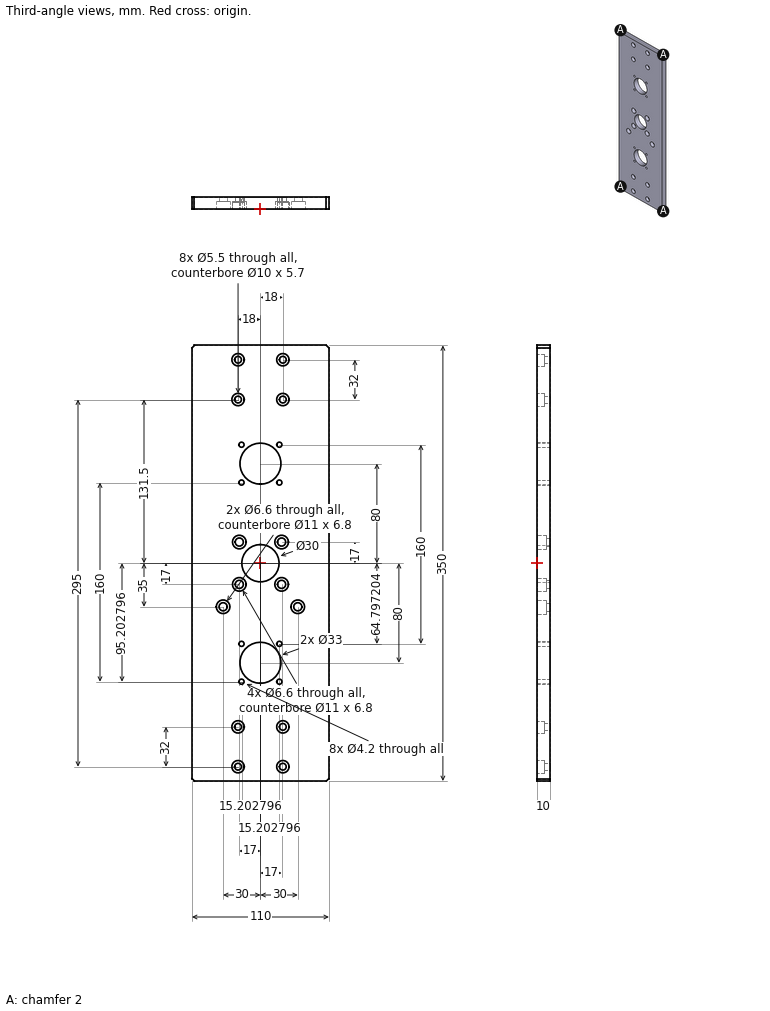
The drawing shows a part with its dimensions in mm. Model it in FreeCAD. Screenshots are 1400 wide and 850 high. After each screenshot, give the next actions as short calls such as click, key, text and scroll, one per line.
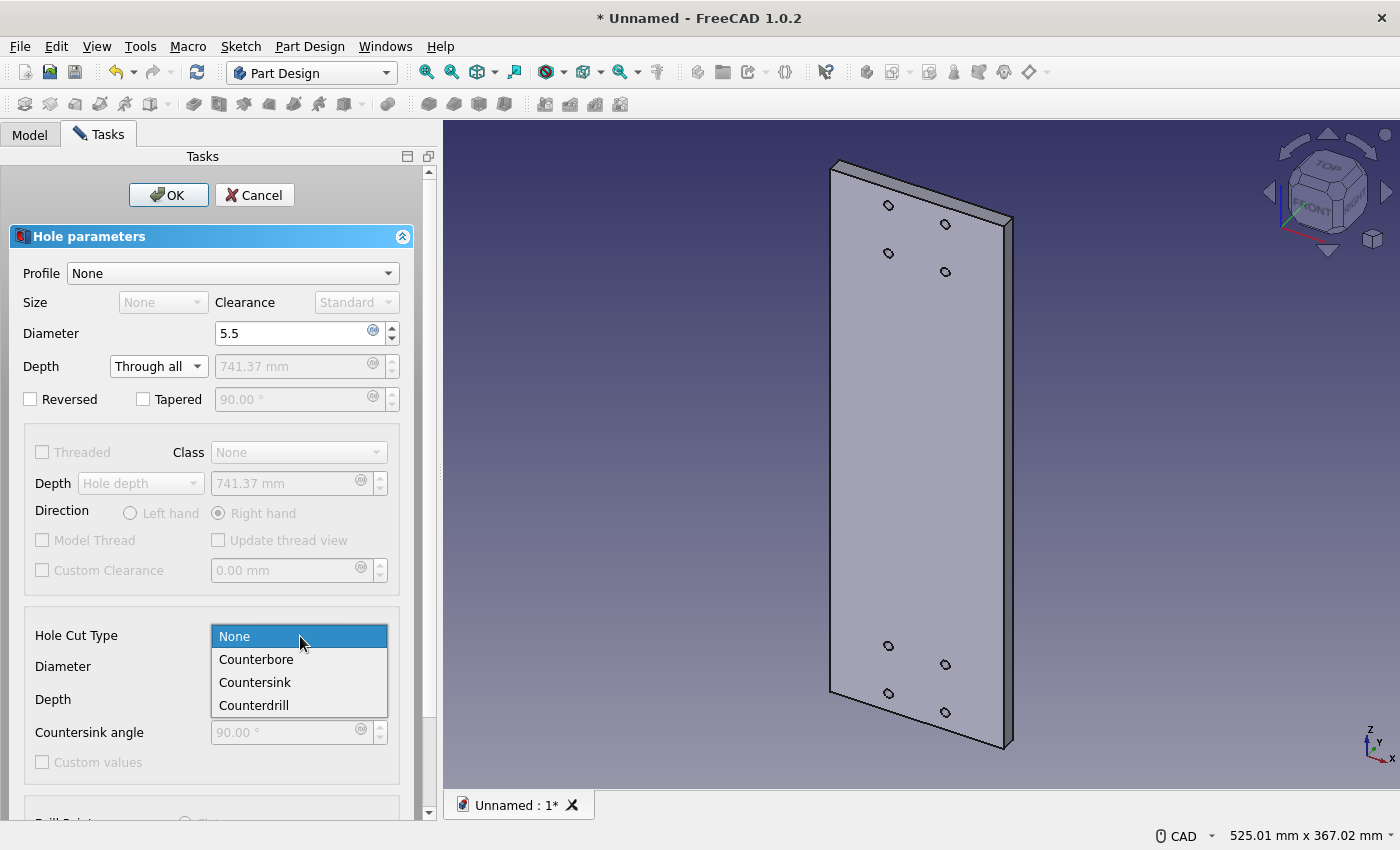
click(298, 660)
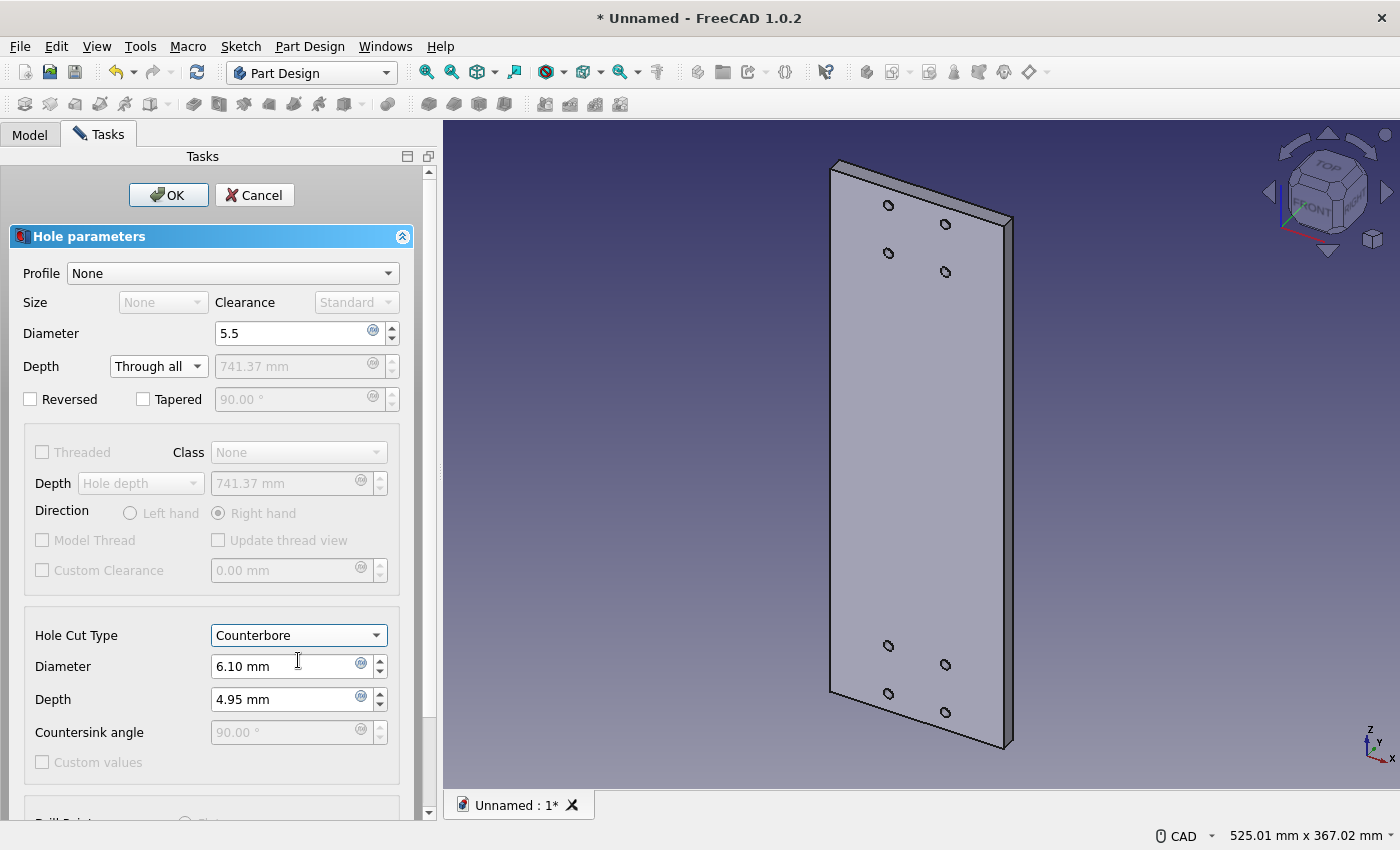
triple_click(292, 666)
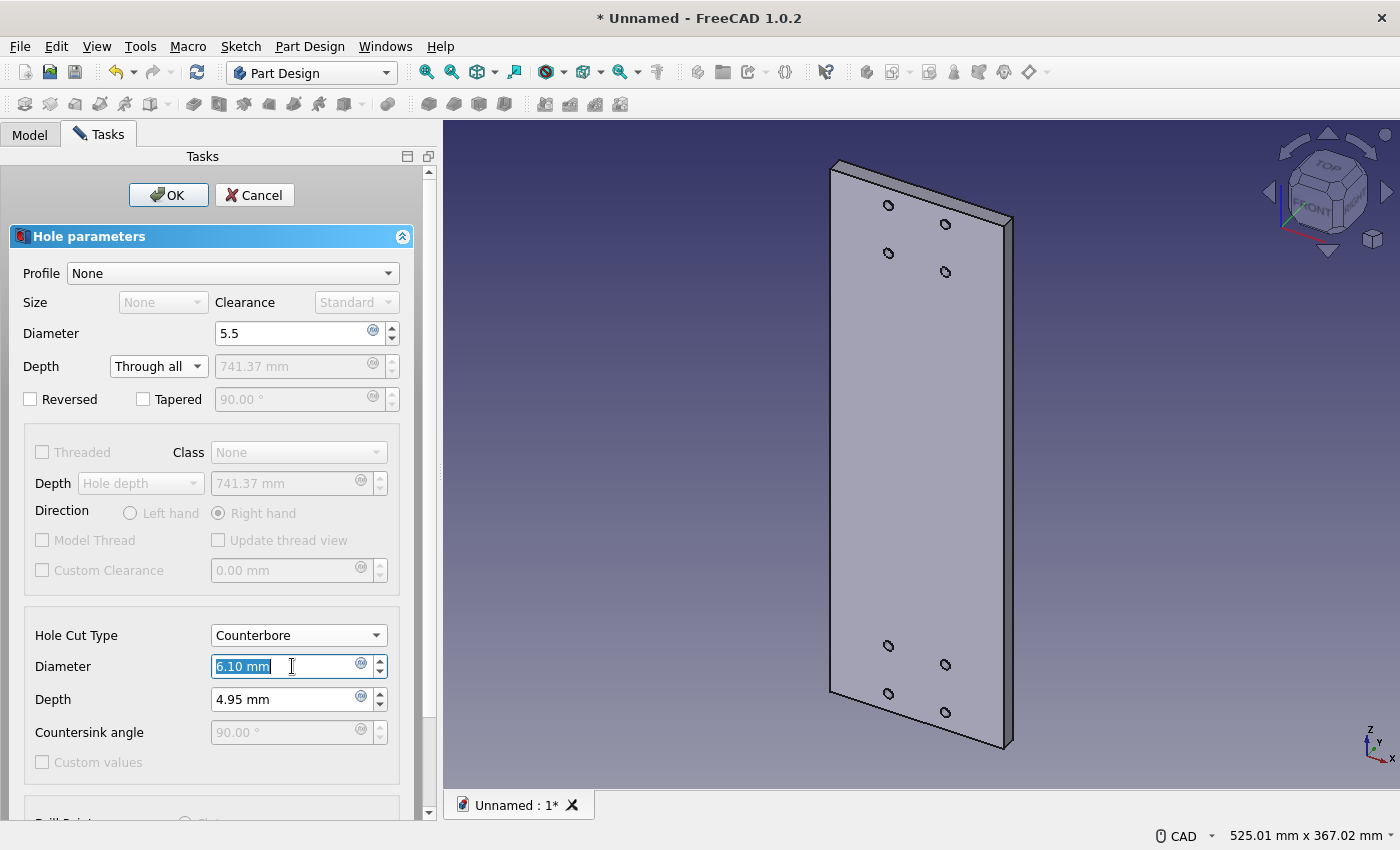
text(10)
key(Tab)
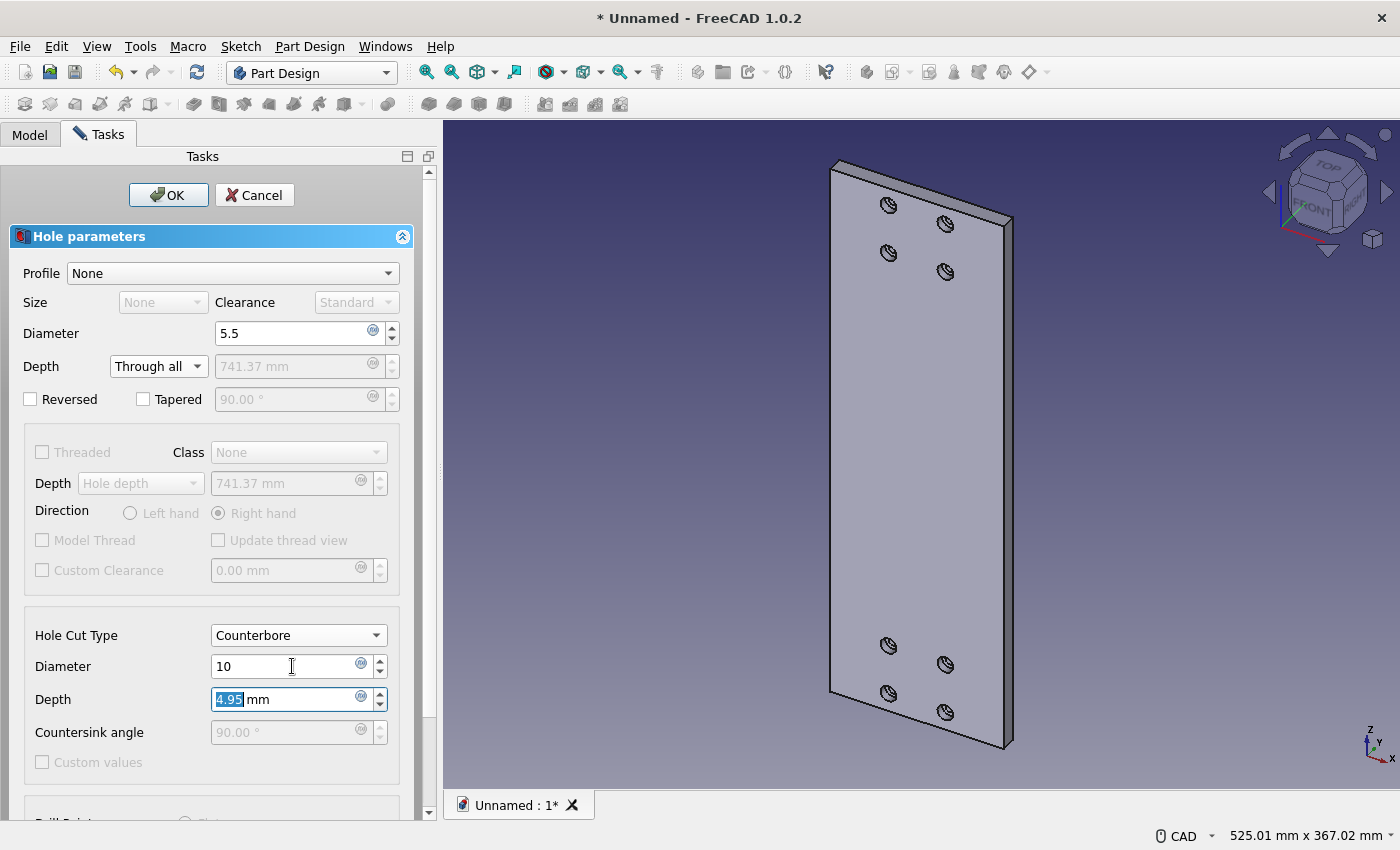
text(5.7)
key(Tab)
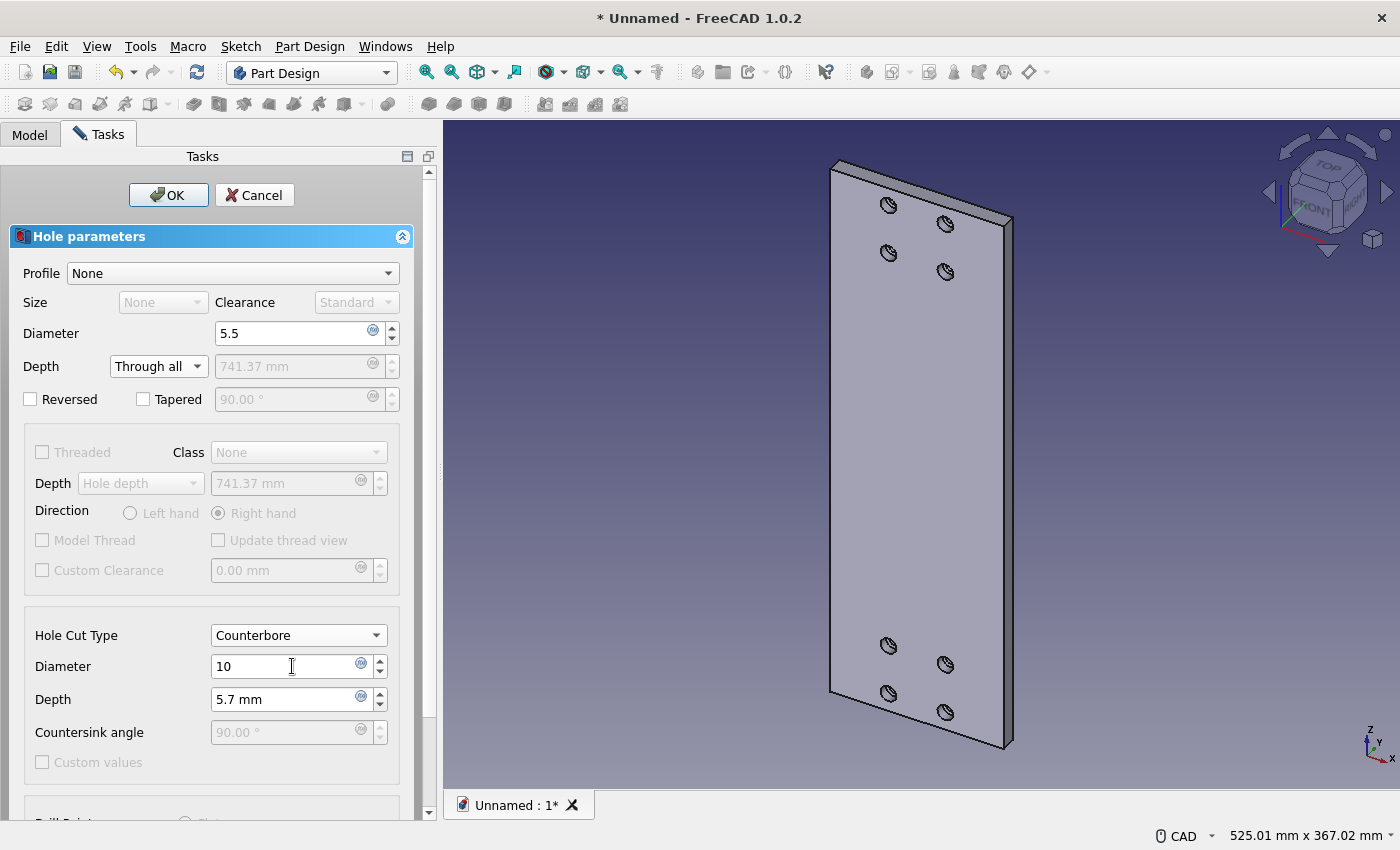
click(169, 195)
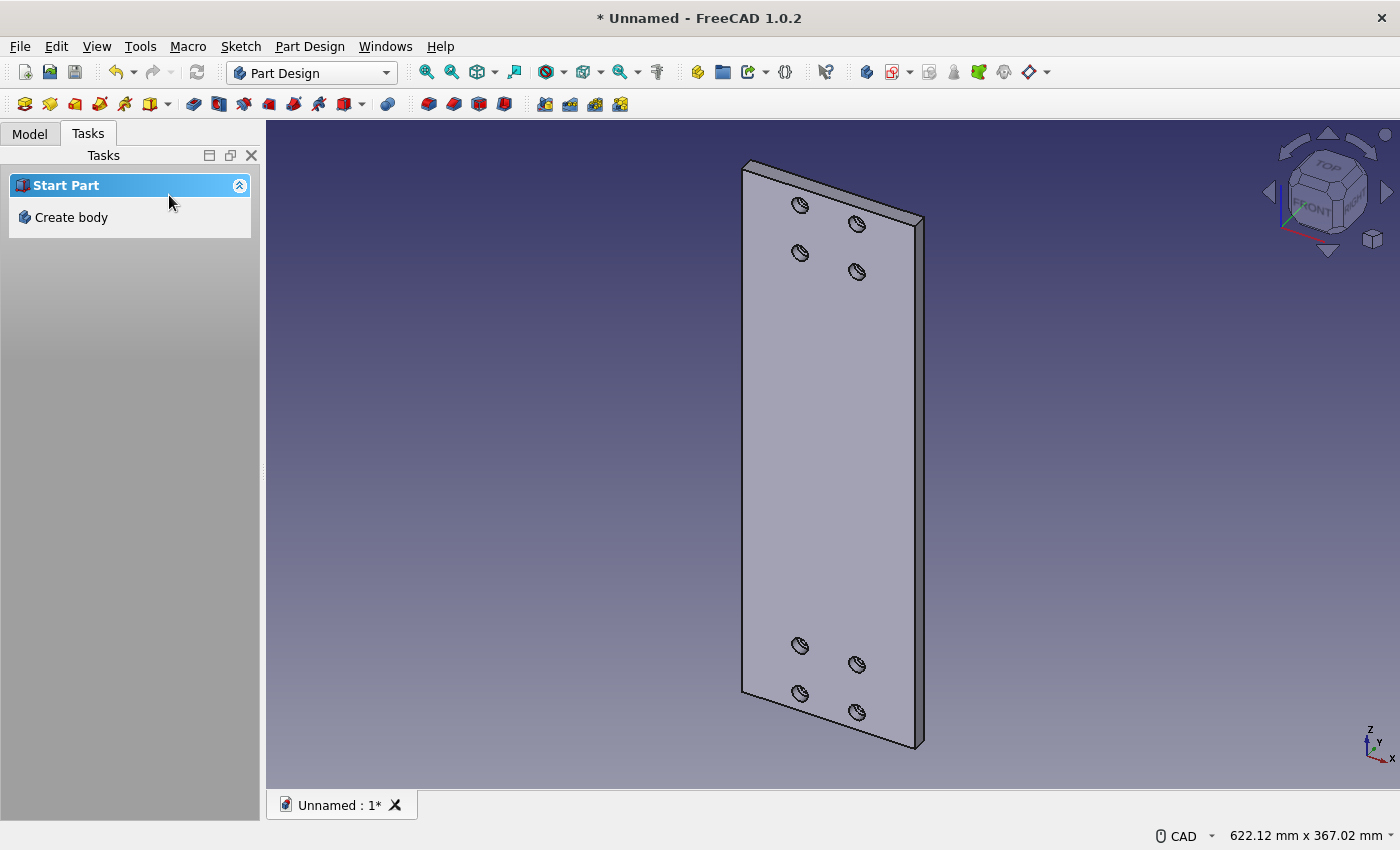
click(828, 383)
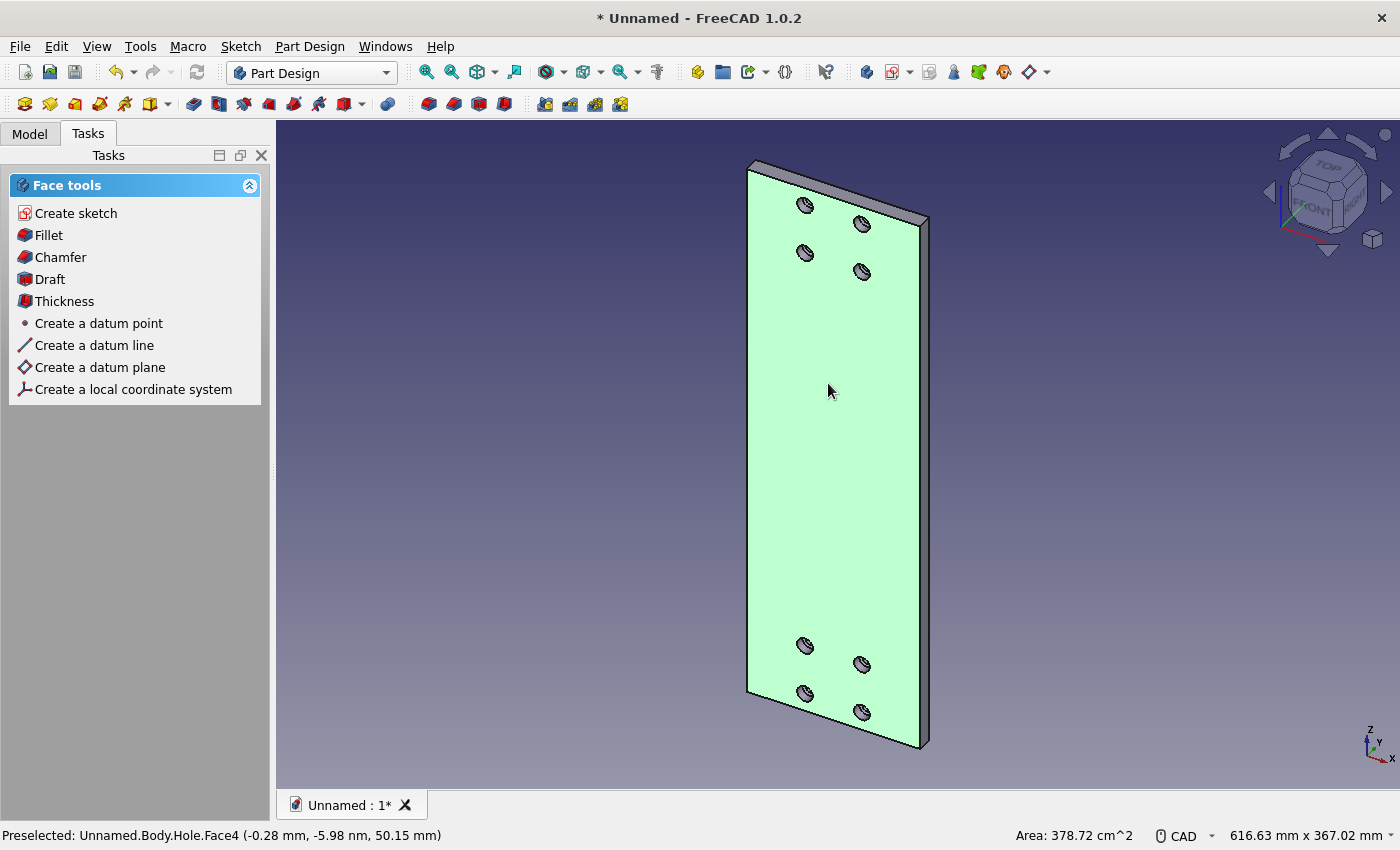
click(892, 72)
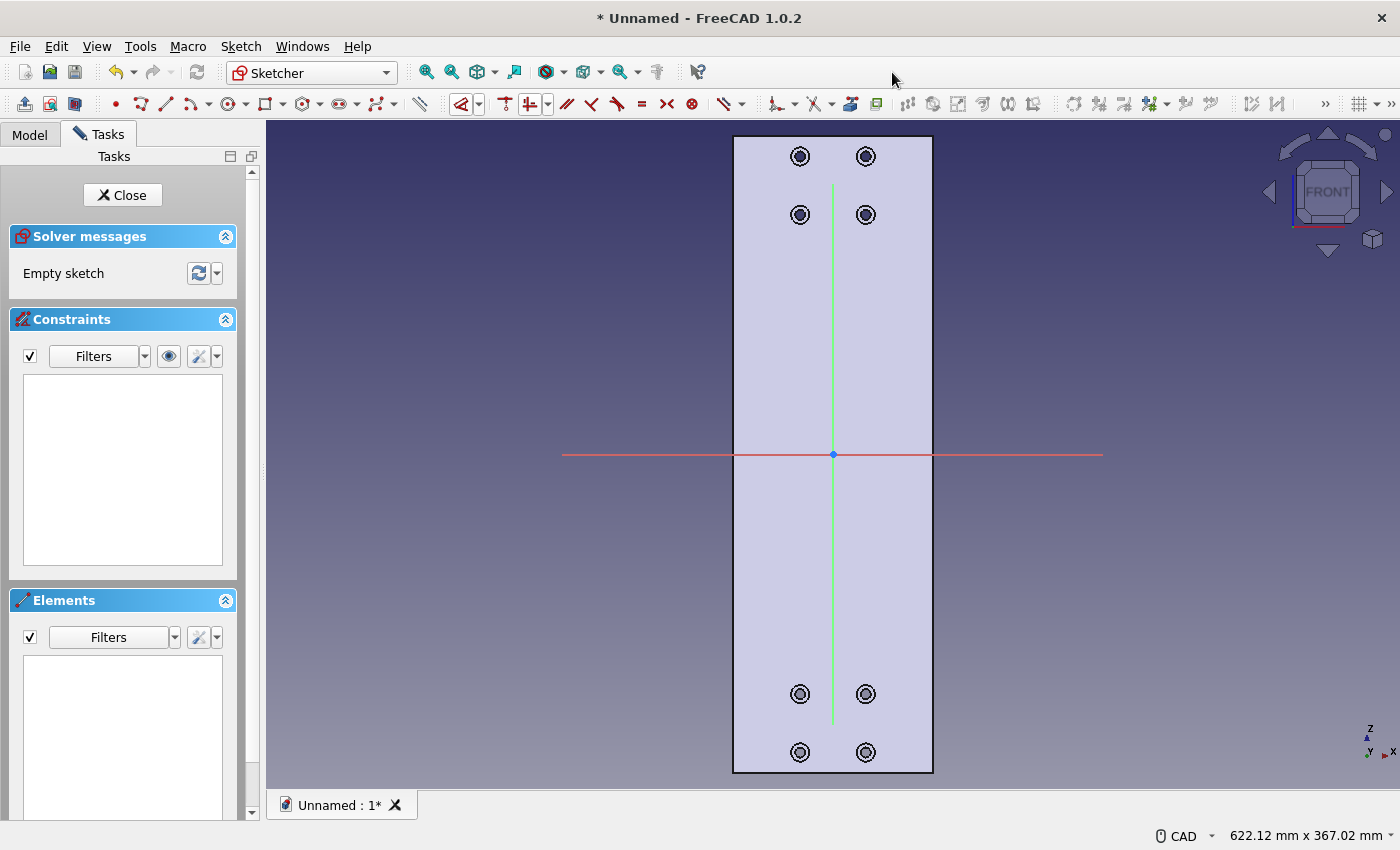
scroll(847, 455, up, 9)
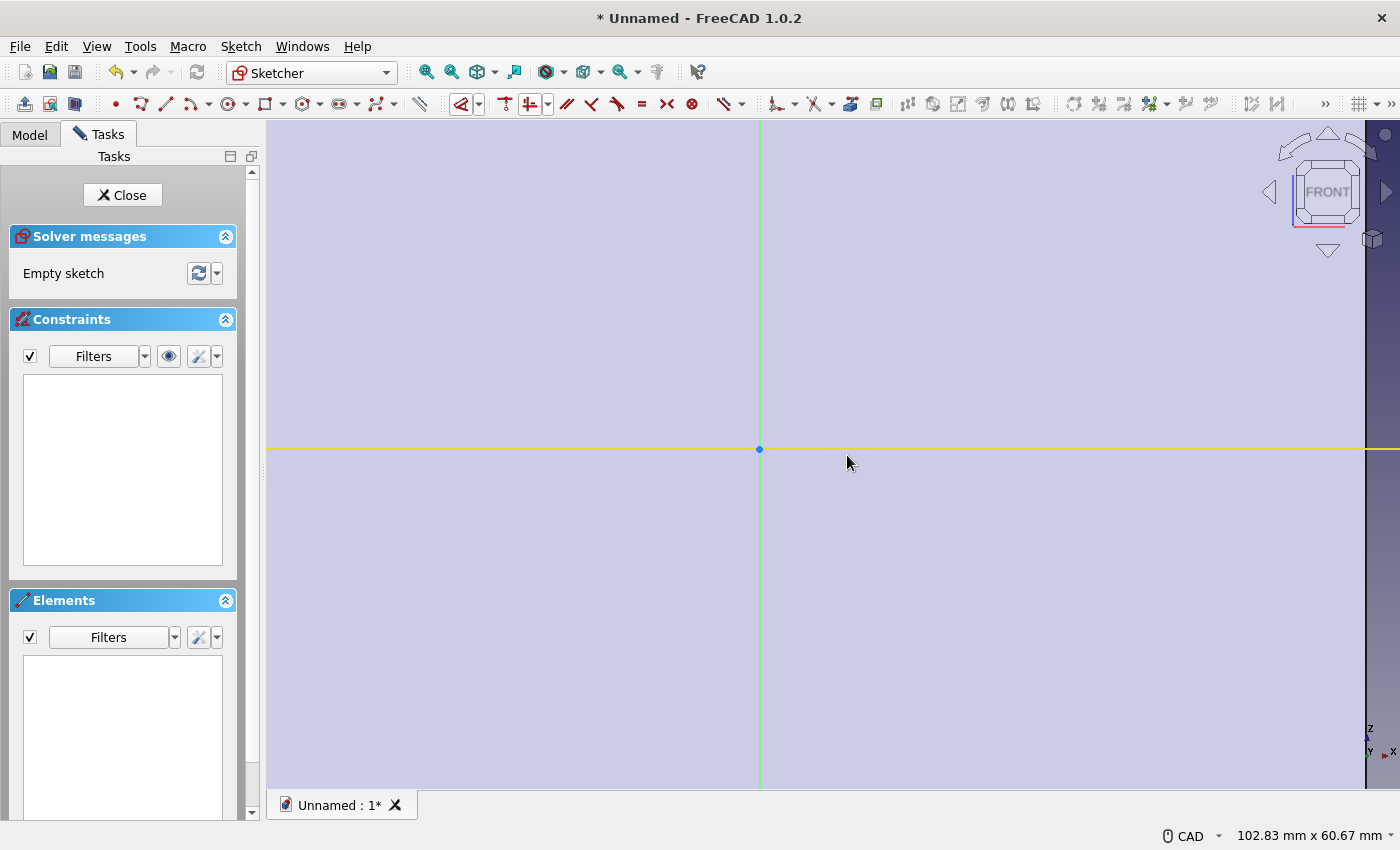
key(g)
key(c)